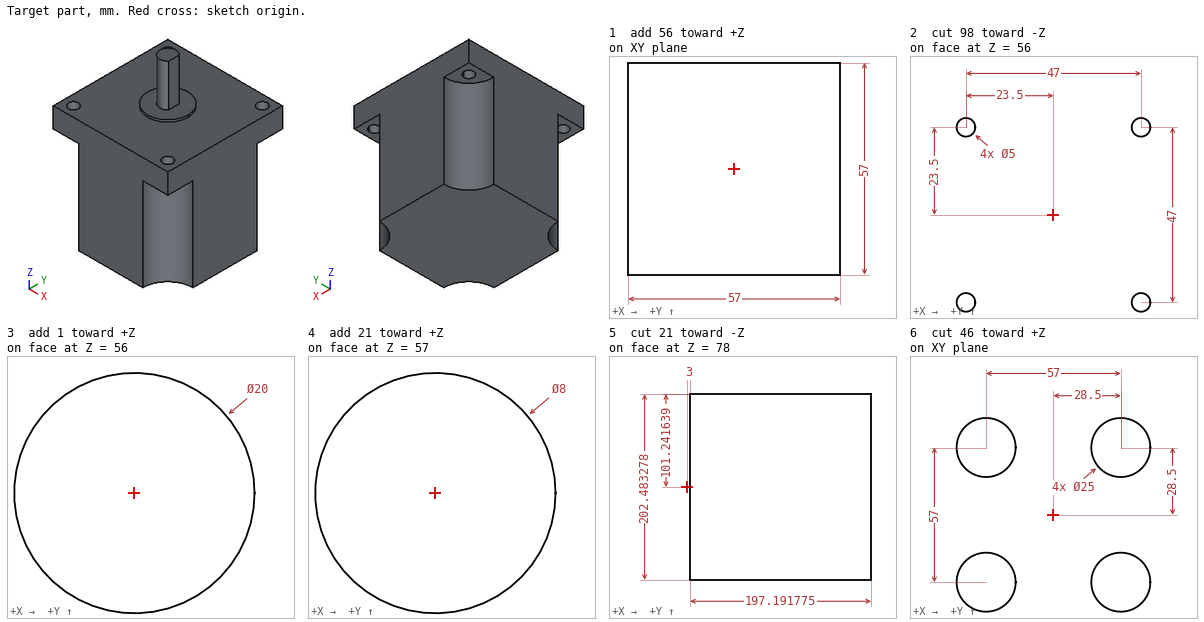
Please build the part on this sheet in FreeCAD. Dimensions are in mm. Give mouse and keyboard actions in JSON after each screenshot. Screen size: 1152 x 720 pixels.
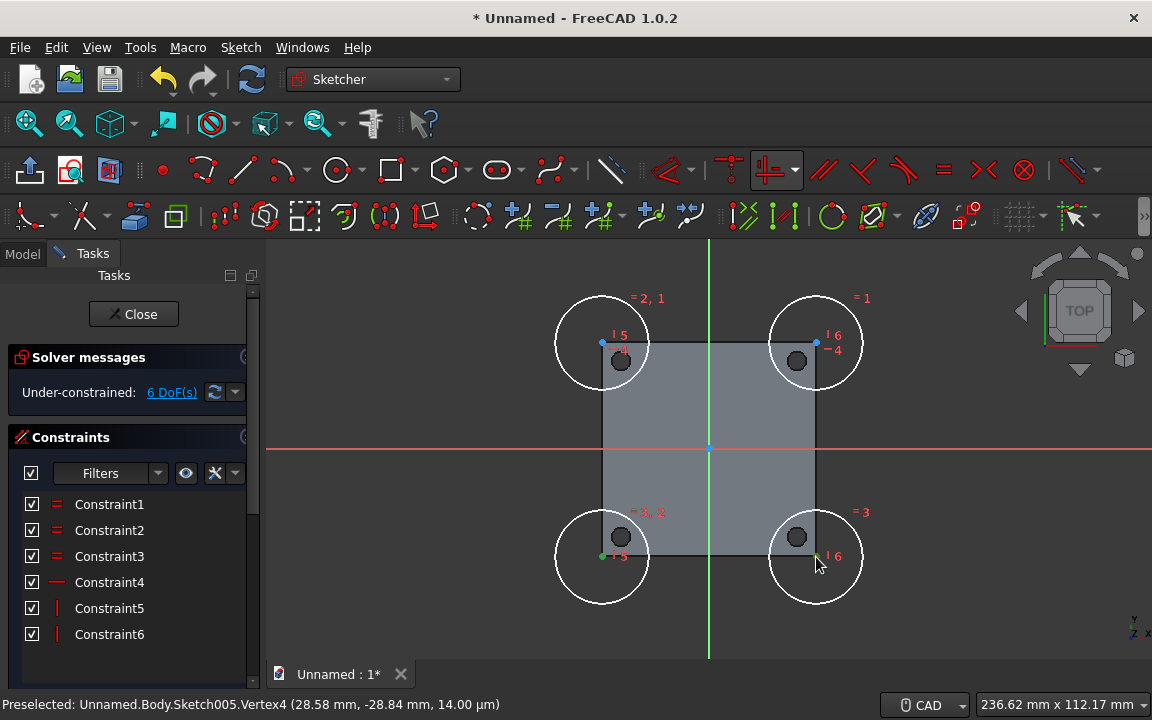
{"action": "key", "text": "h"}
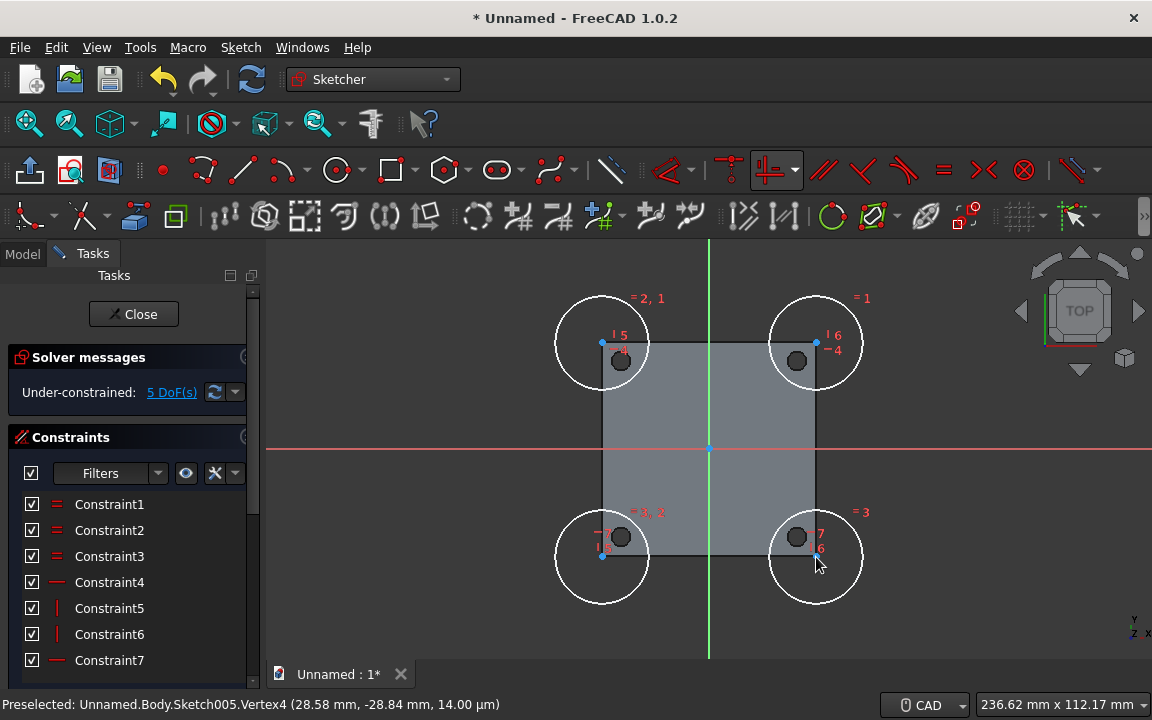
{"action": "left_click", "coordinate": [666, 170]}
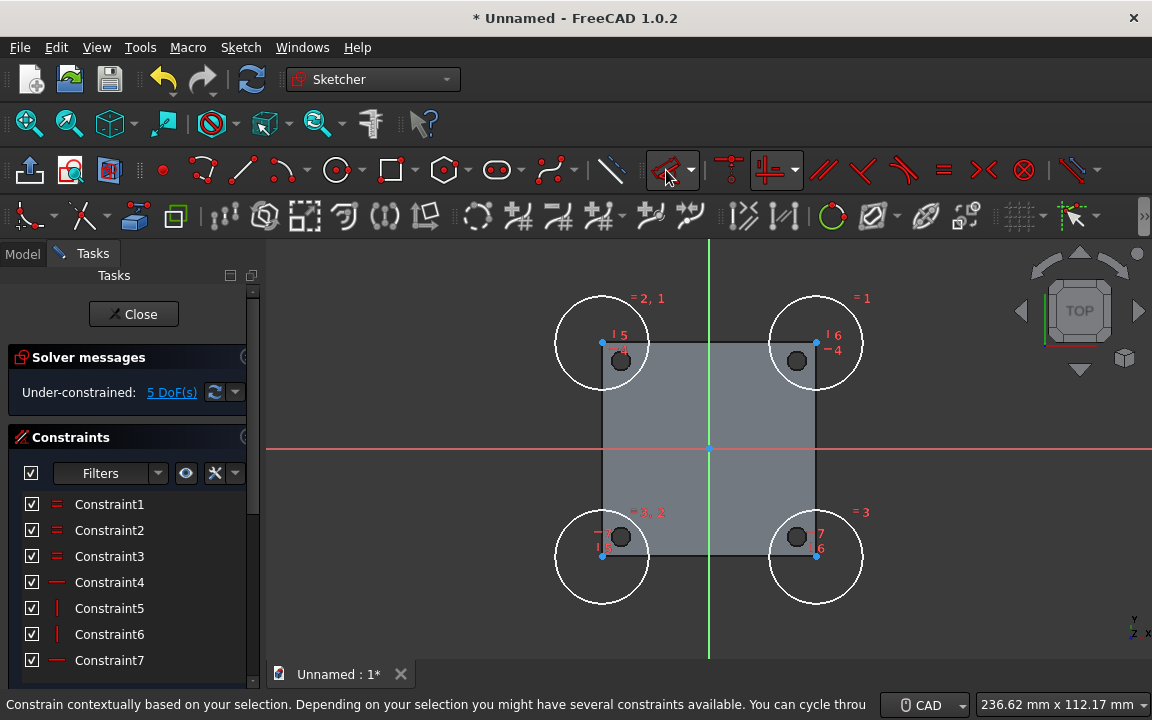
{"action": "left_click", "coordinate": [849, 310]}
{"action": "left_click", "coordinate": [872, 287]}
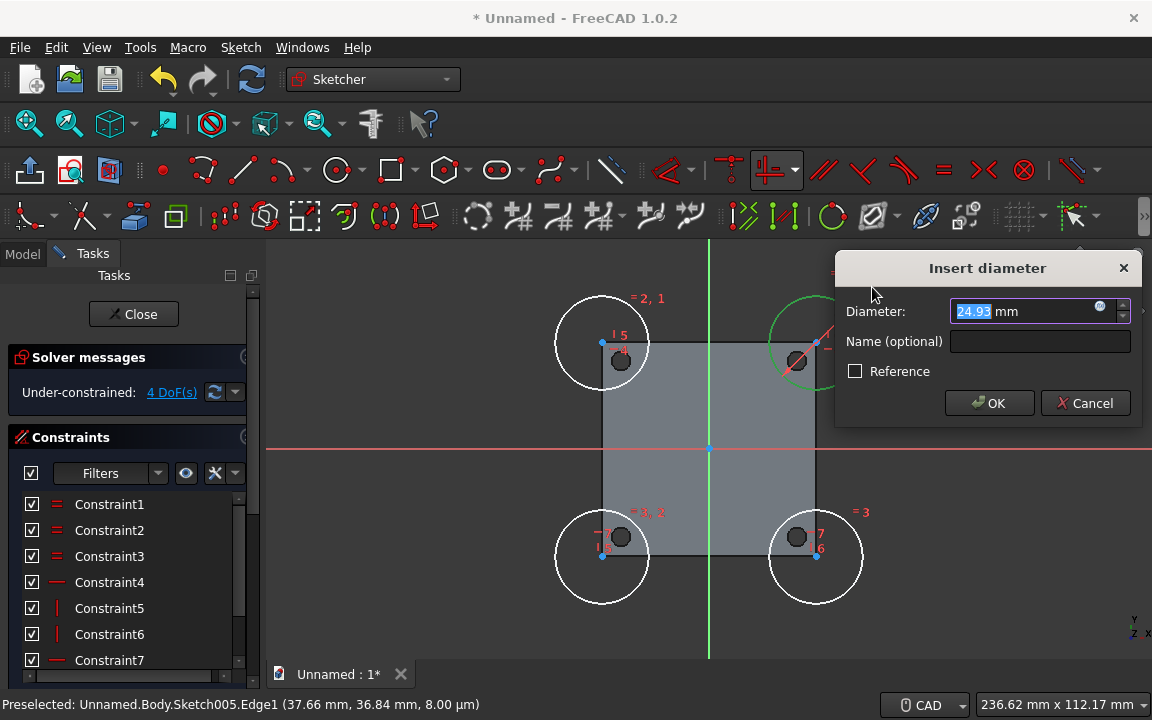
{"action": "type", "text": "25"}
{"action": "key", "text": "Return"}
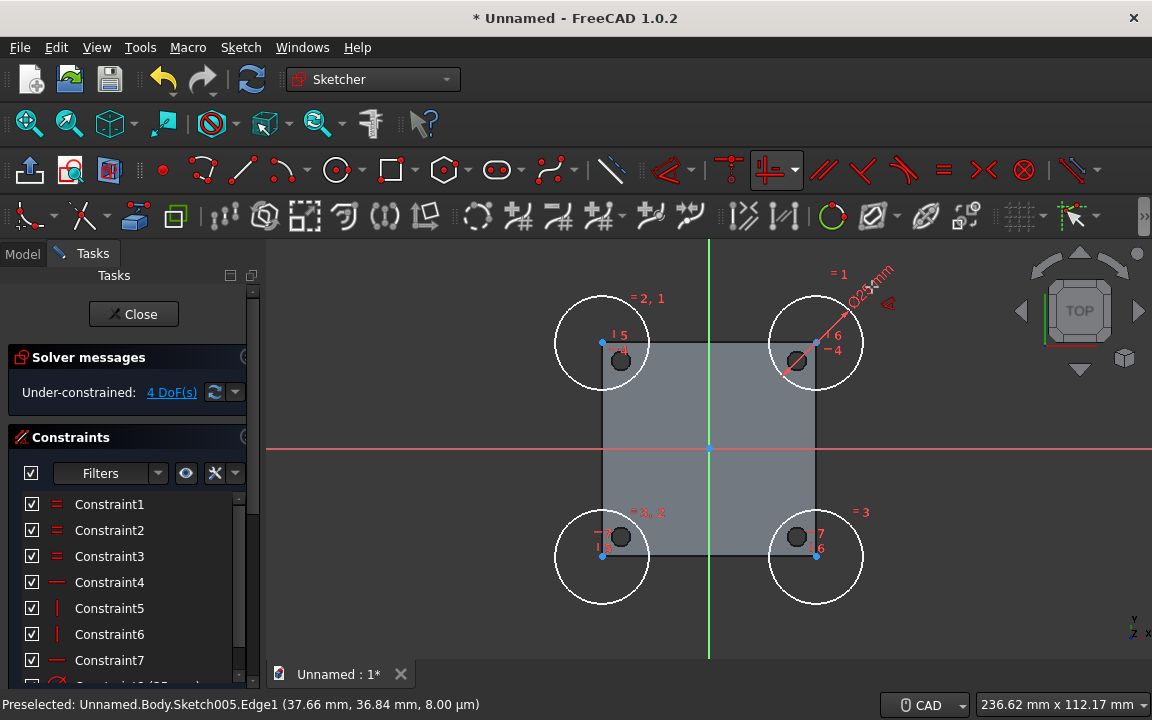
{"action": "left_click", "coordinate": [816, 343]}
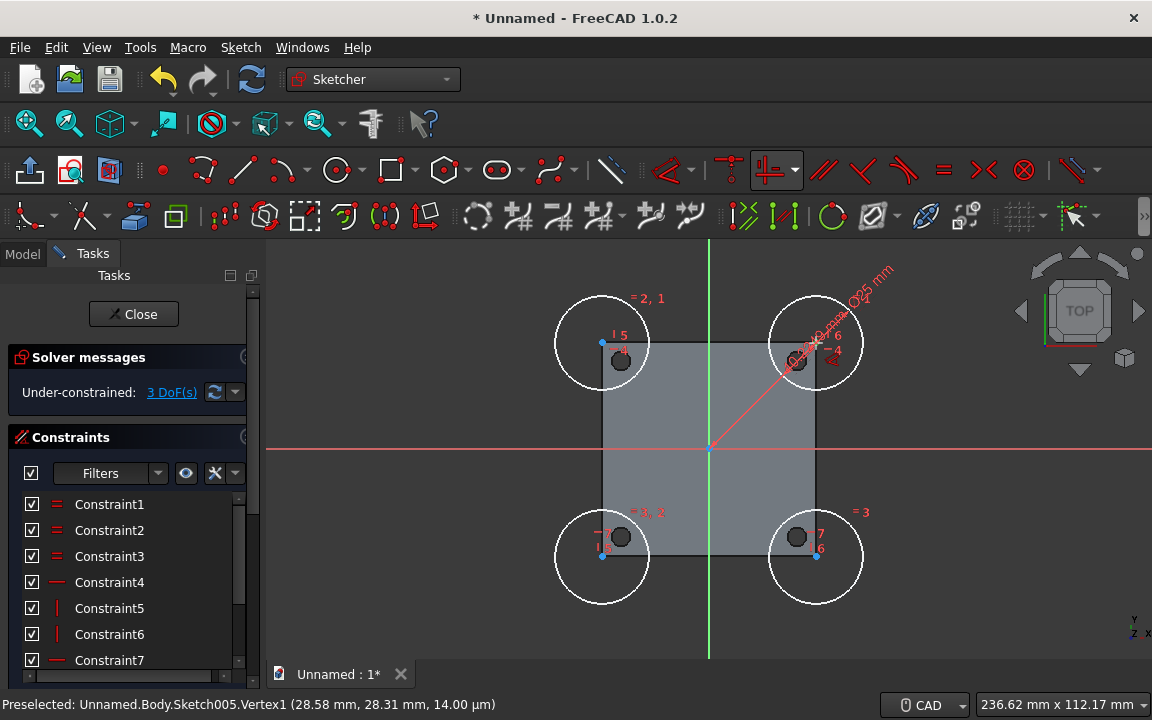
{"action": "left_click", "coordinate": [602, 343]}
{"action": "left_click", "coordinate": [660, 309]}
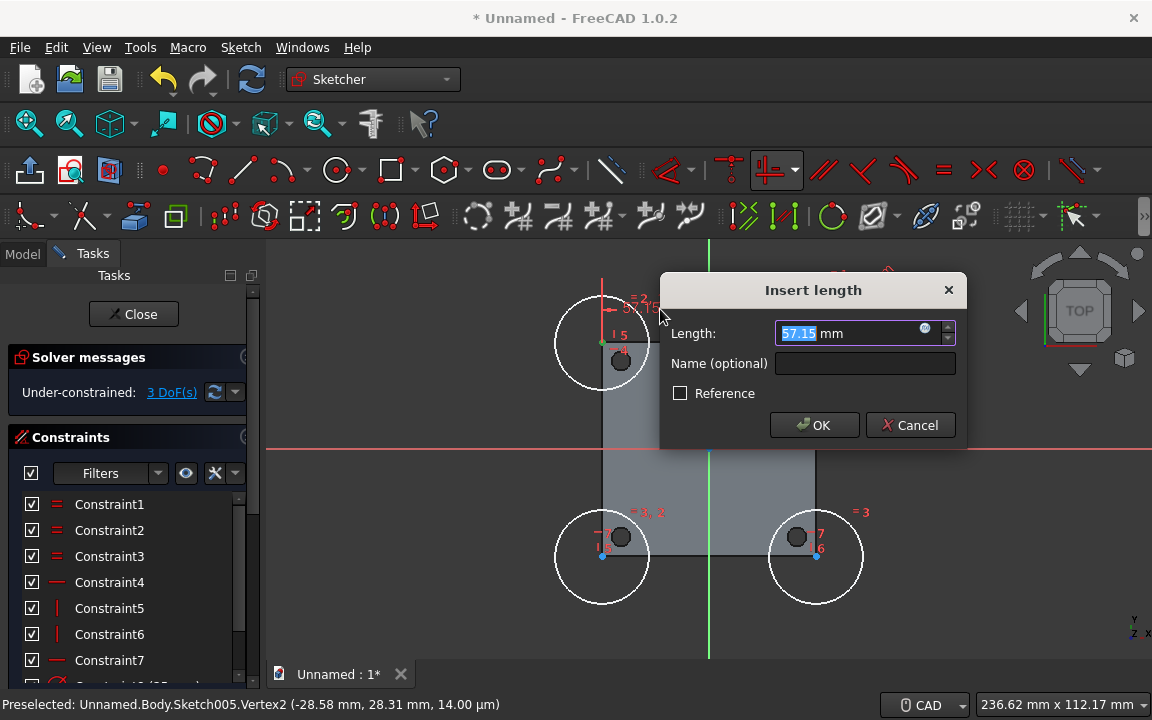
{"action": "type", "text": "57"}
{"action": "key", "text": "Return"}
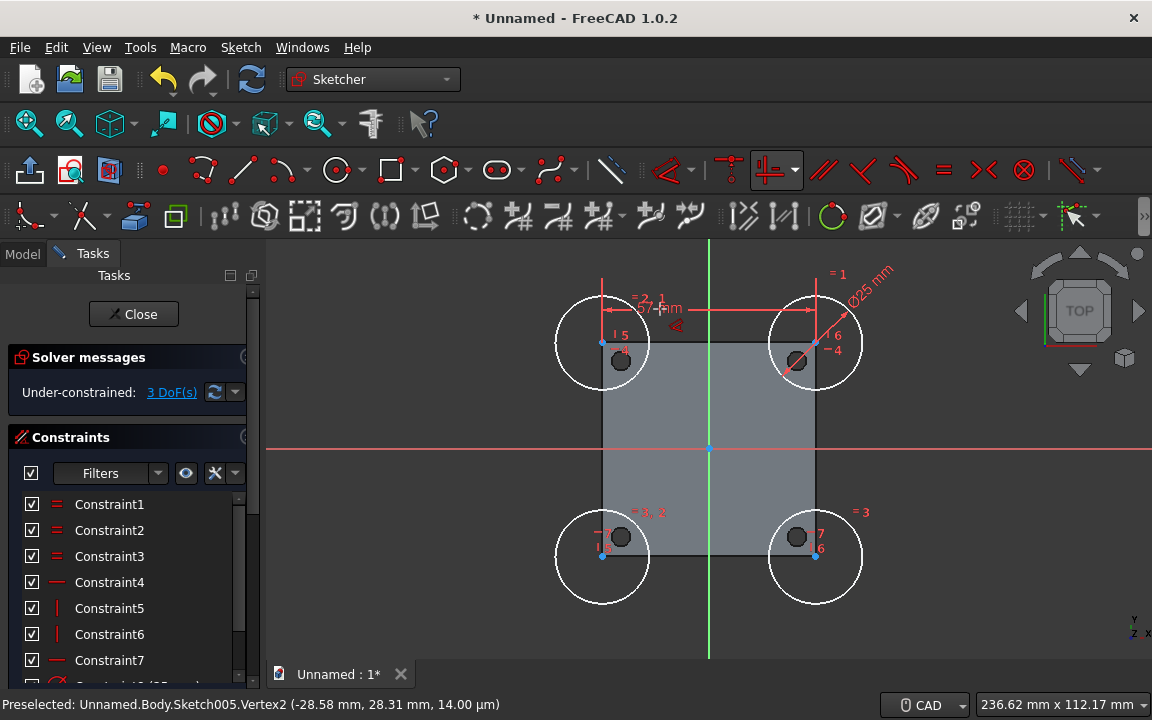
{"action": "left_click", "coordinate": [602, 343]}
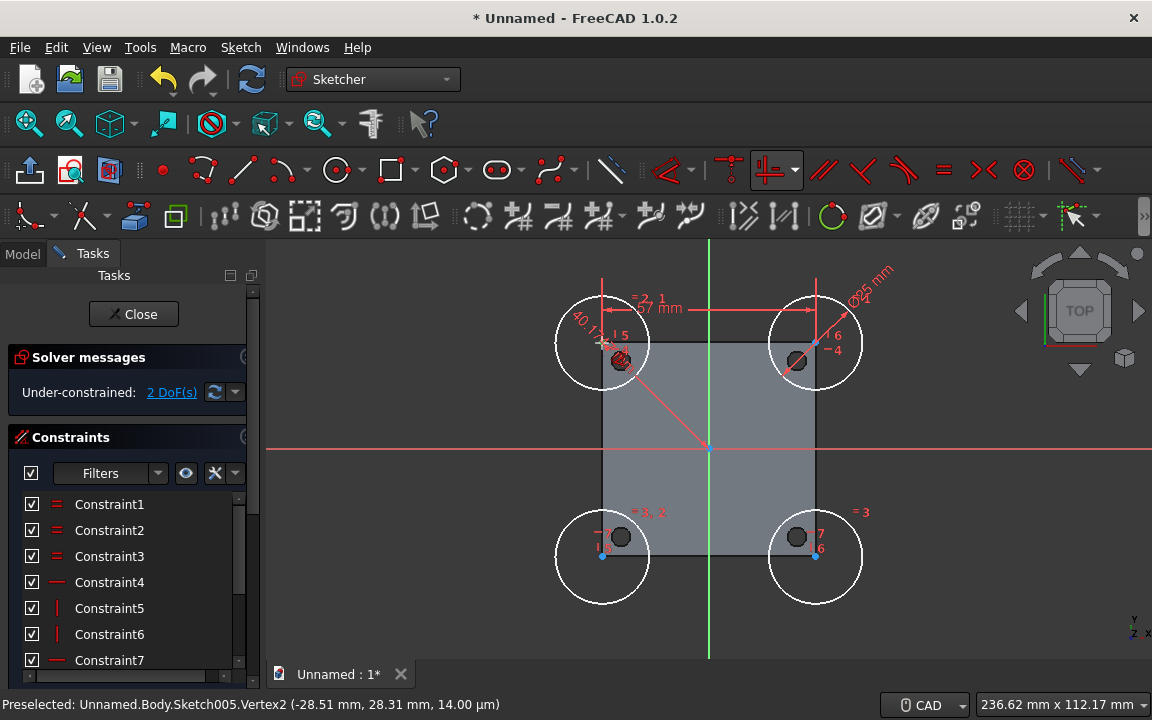
{"action": "left_click", "coordinate": [602, 557]}
{"action": "left_click", "coordinate": [568, 401]}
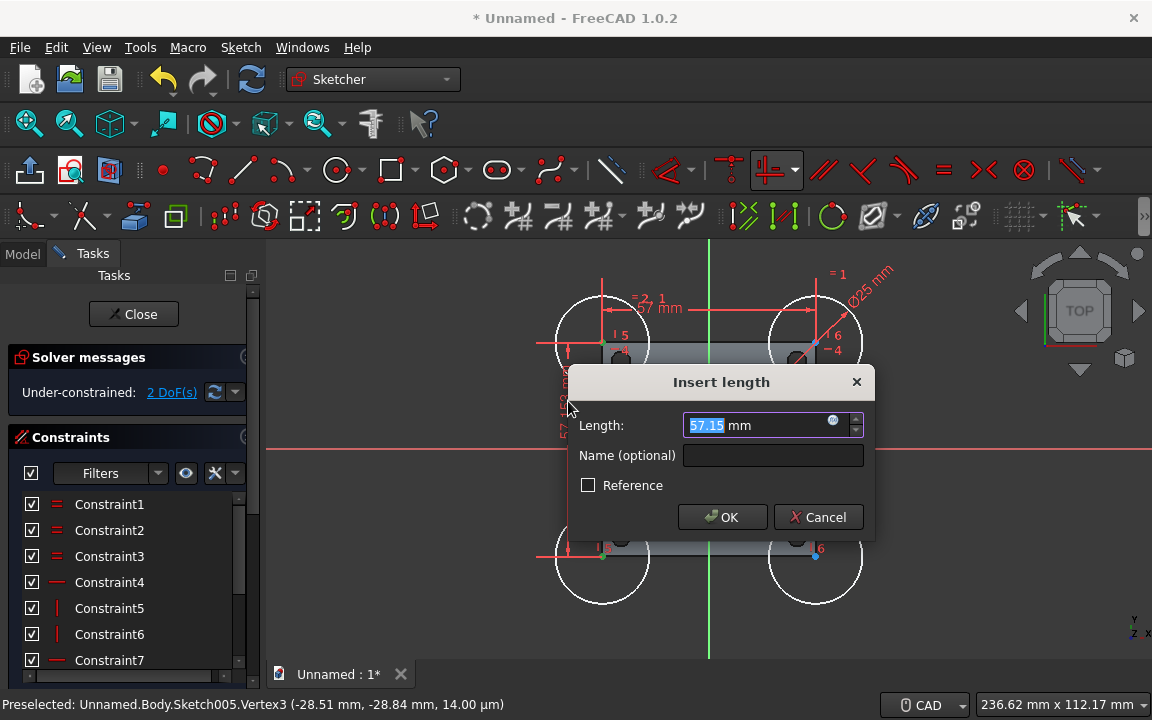
{"action": "type", "text": "57"}
{"action": "key", "text": "Return"}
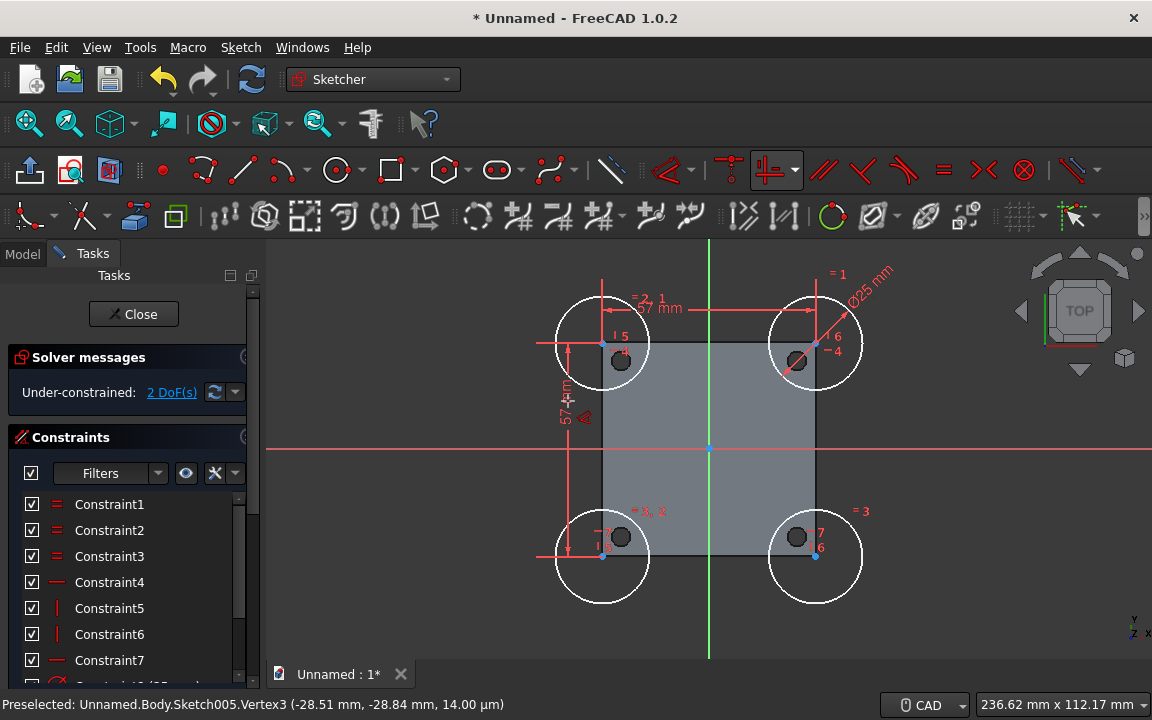
{"action": "left_click", "coordinate": [816, 343]}
{"action": "left_click", "coordinate": [762, 309]}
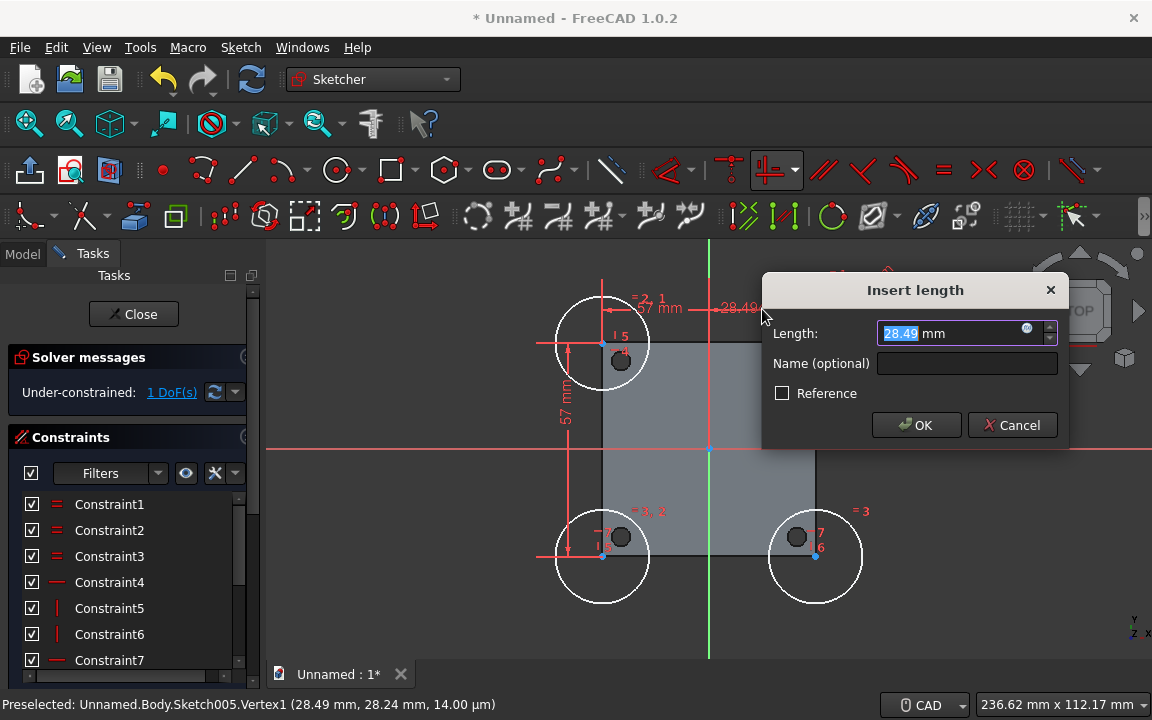
{"action": "type", "text": "28.5"}
{"action": "key", "text": "Return"}